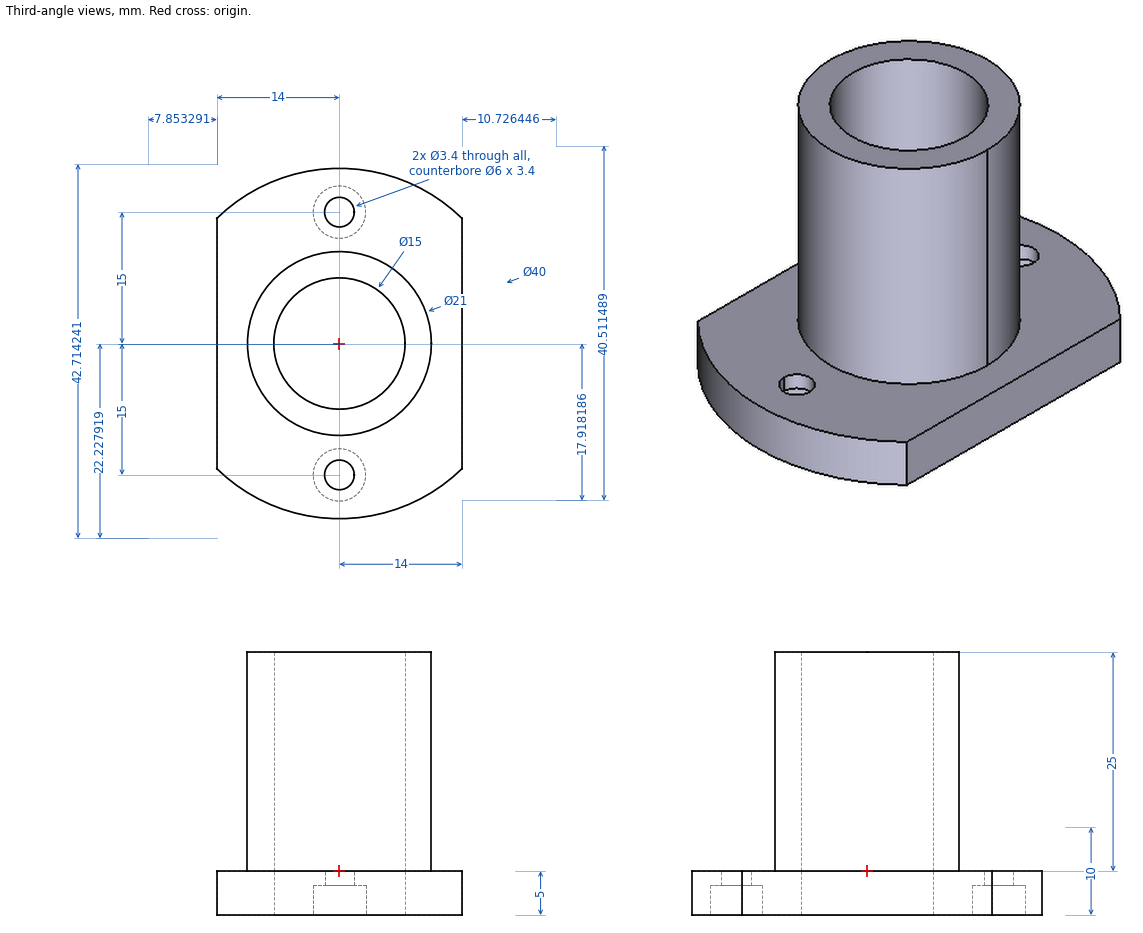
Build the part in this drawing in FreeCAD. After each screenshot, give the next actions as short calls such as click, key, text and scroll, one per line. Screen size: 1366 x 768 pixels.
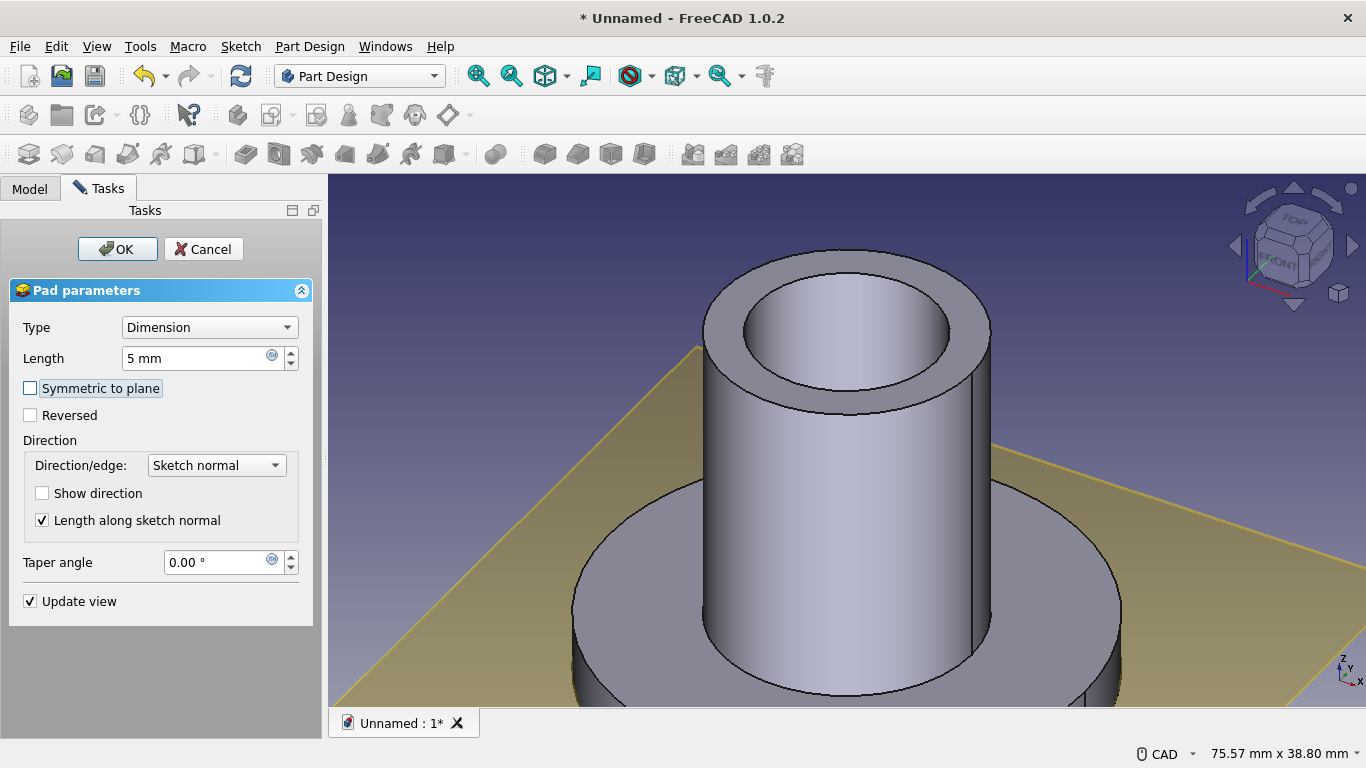
click(118, 249)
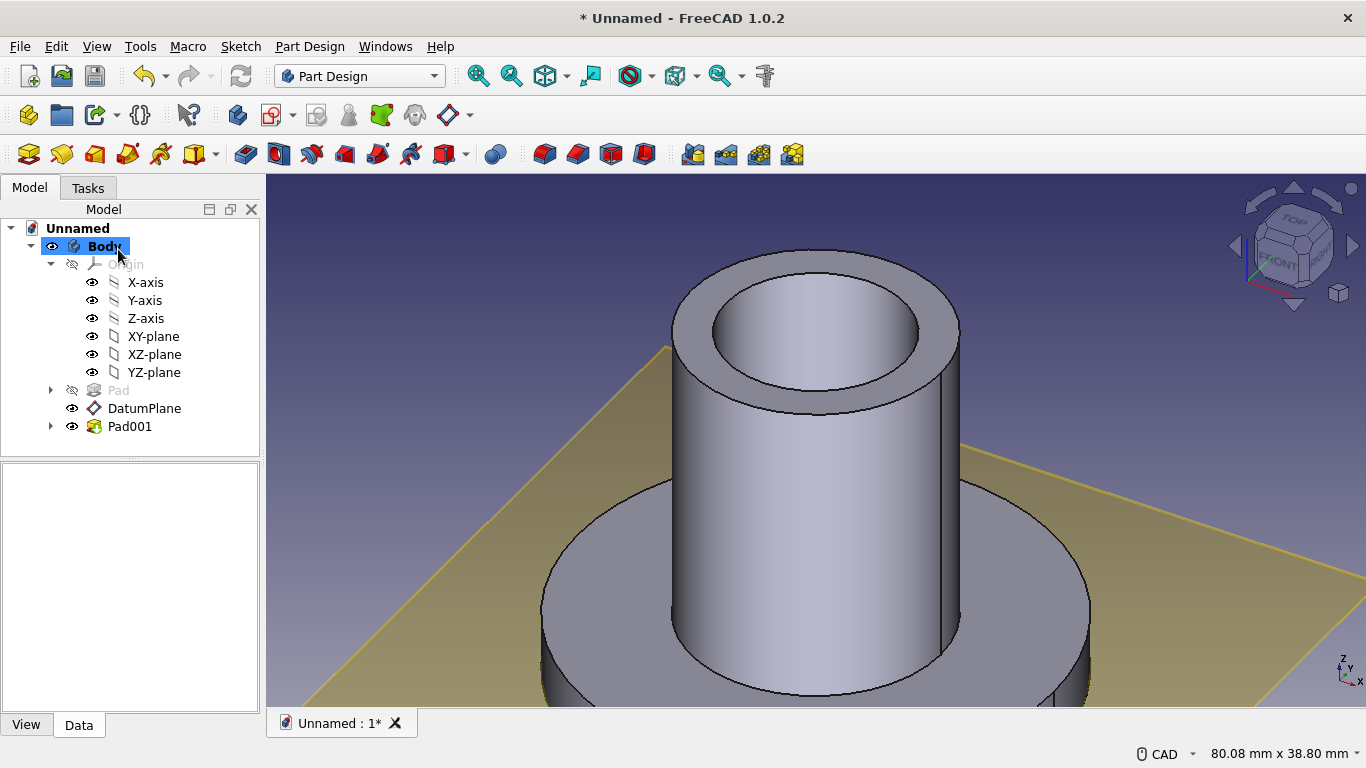
click(117, 408)
key(space)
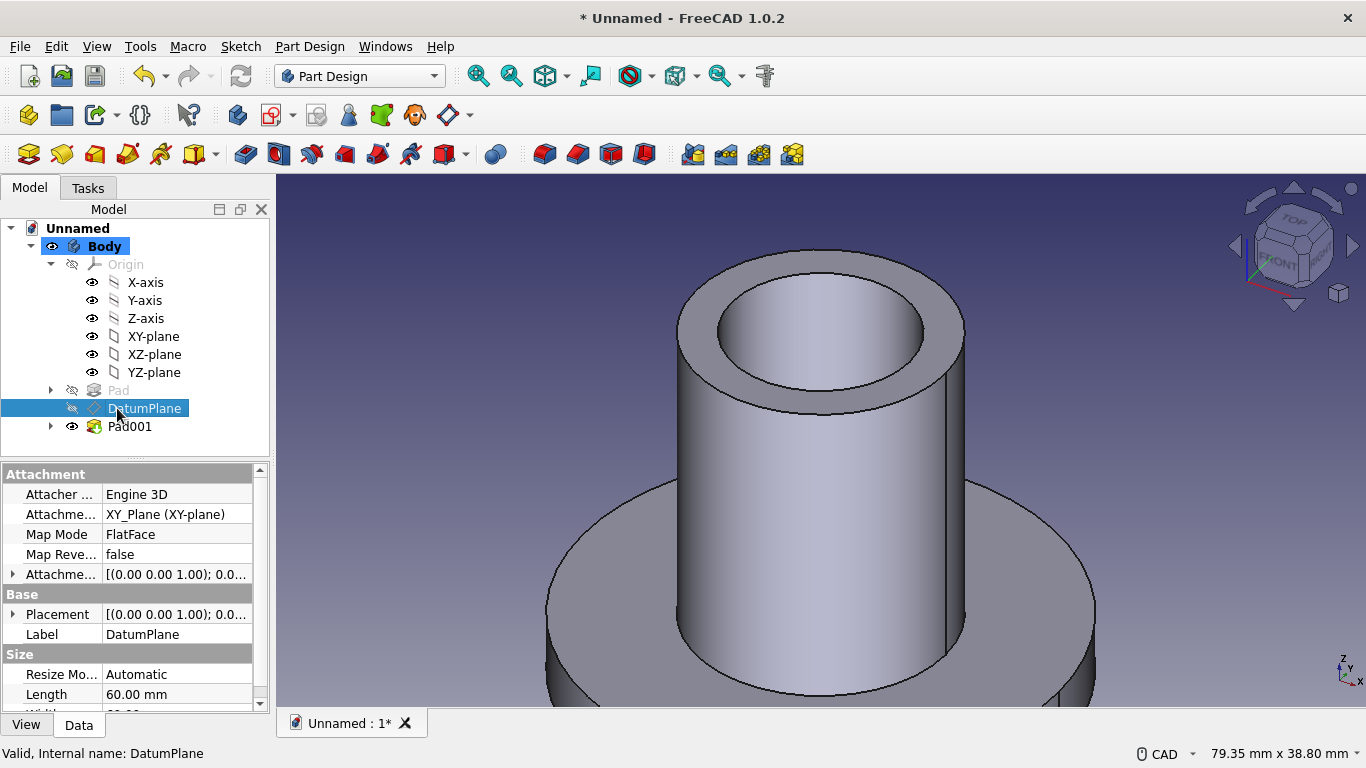
click(479, 76)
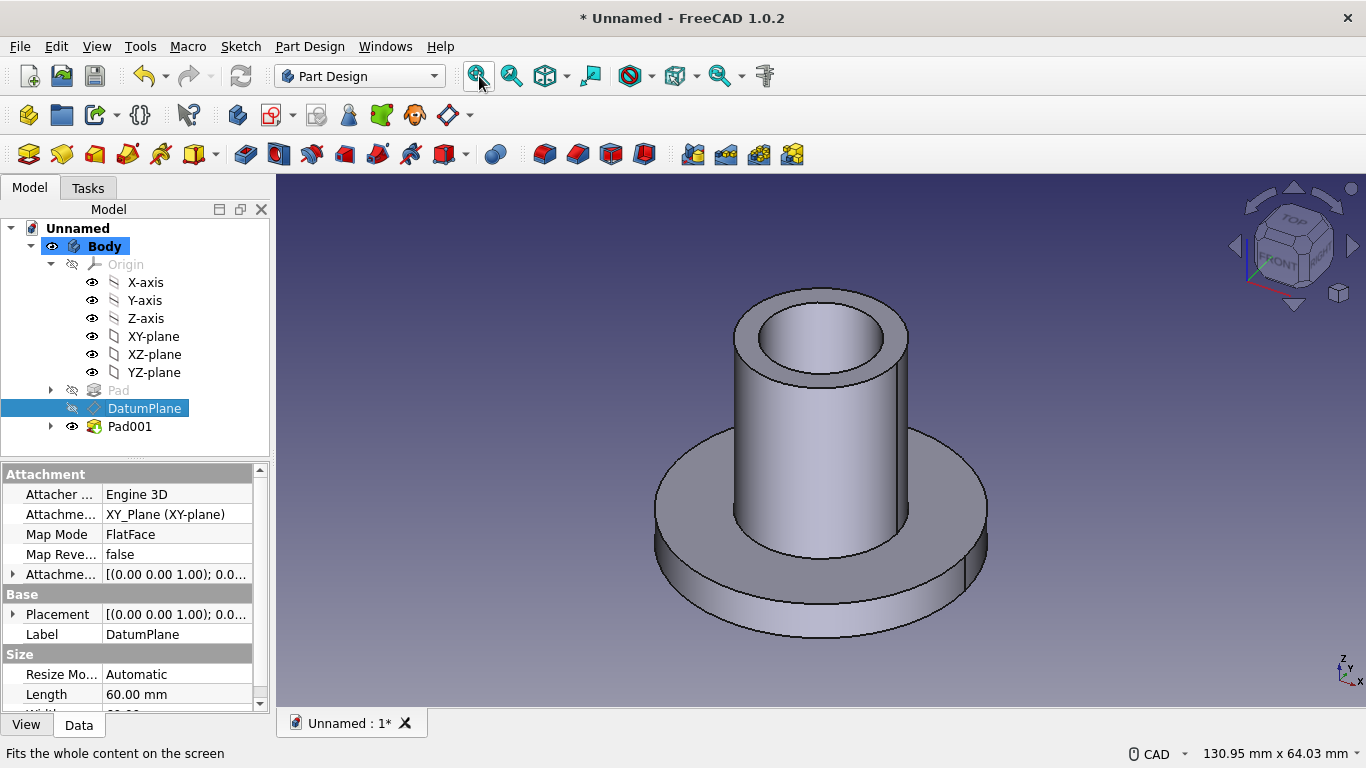
key(5)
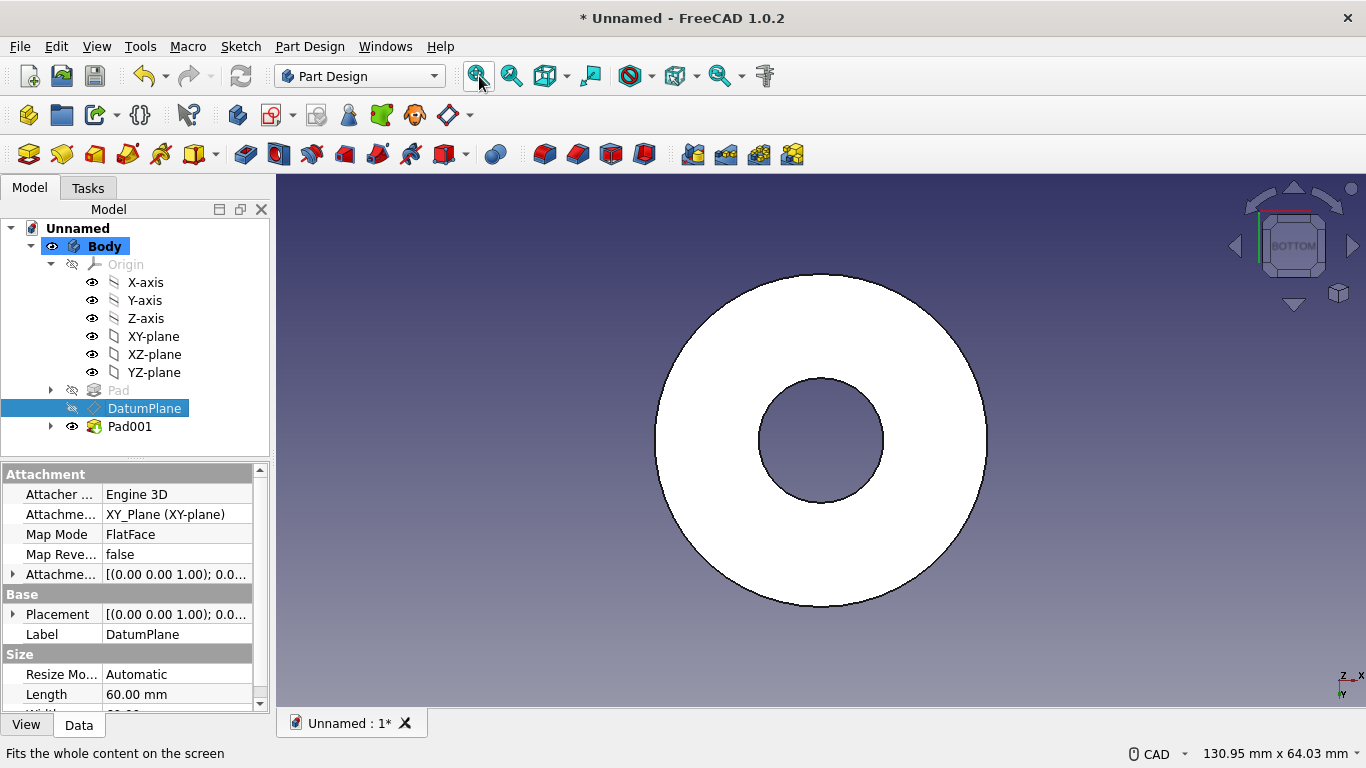
click(726, 487)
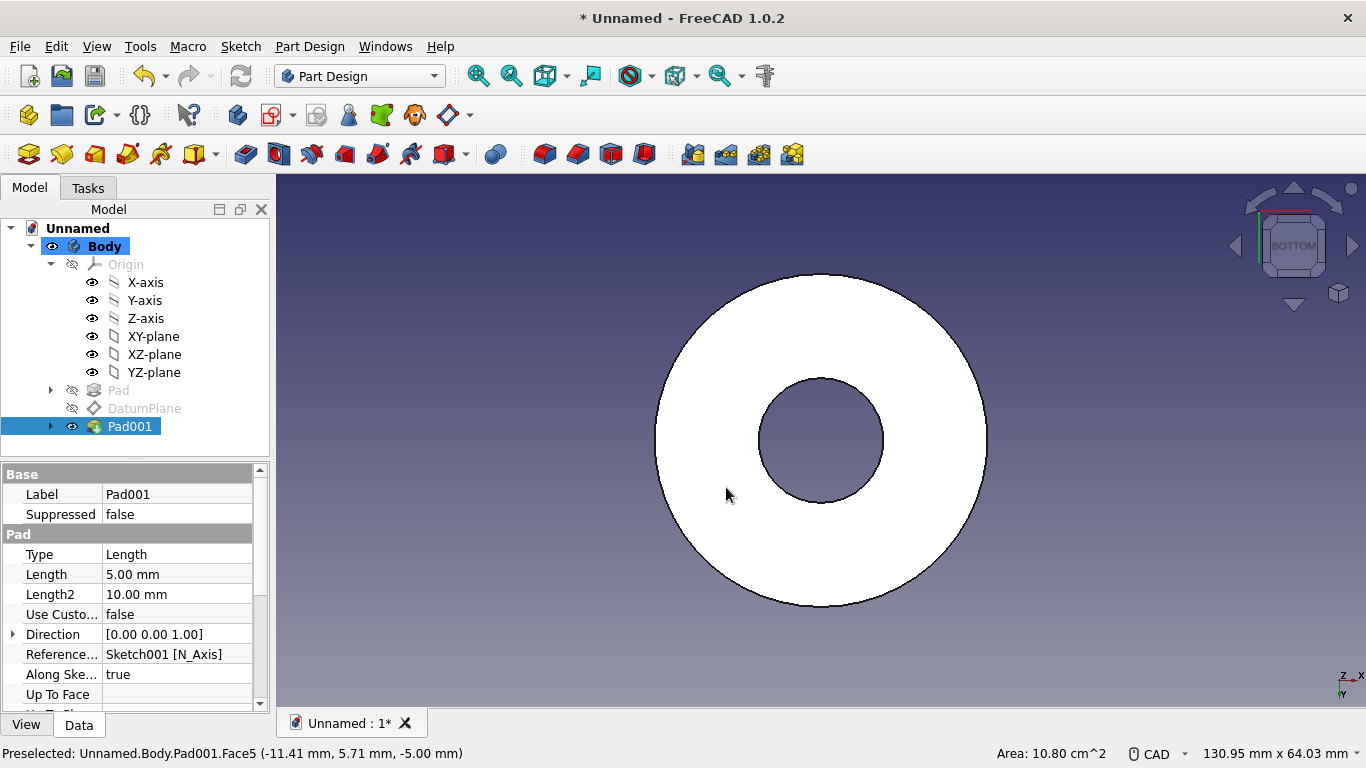
click(270, 116)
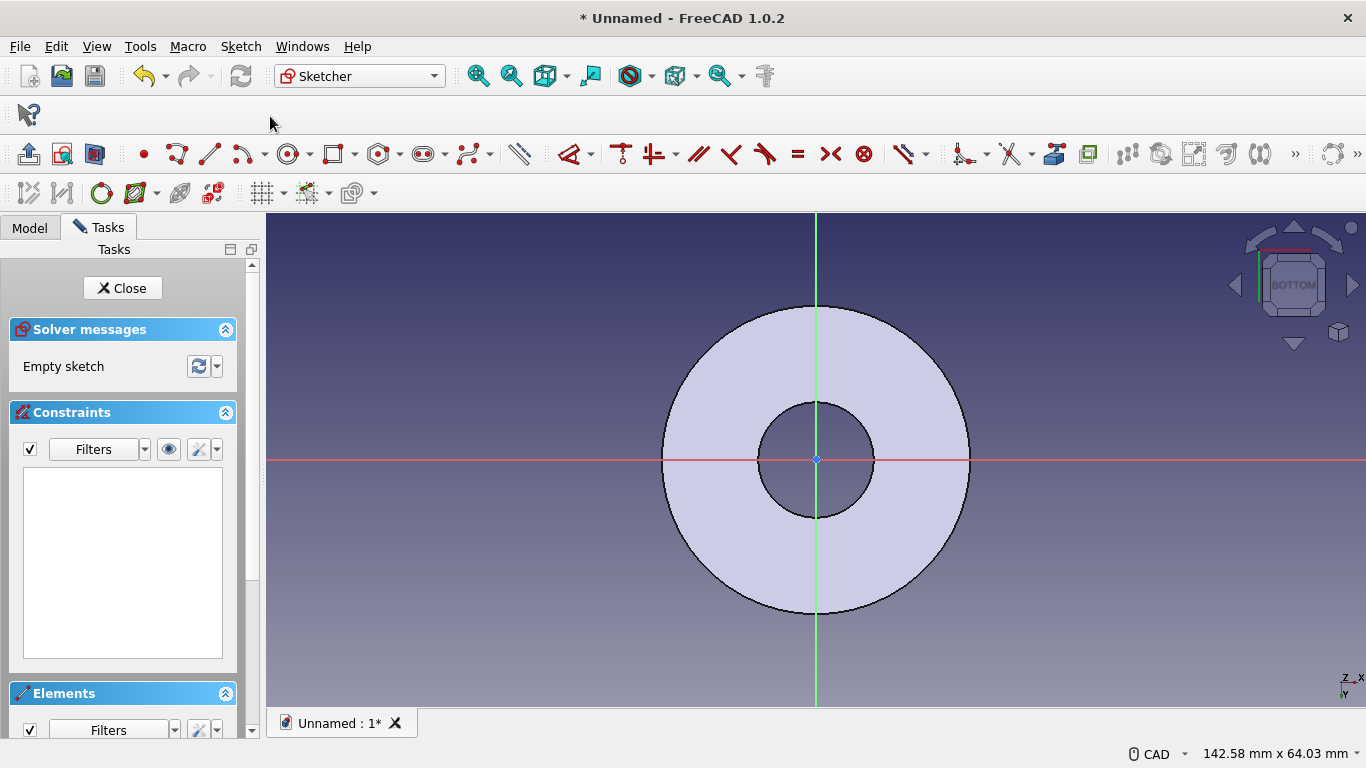
click(288, 154)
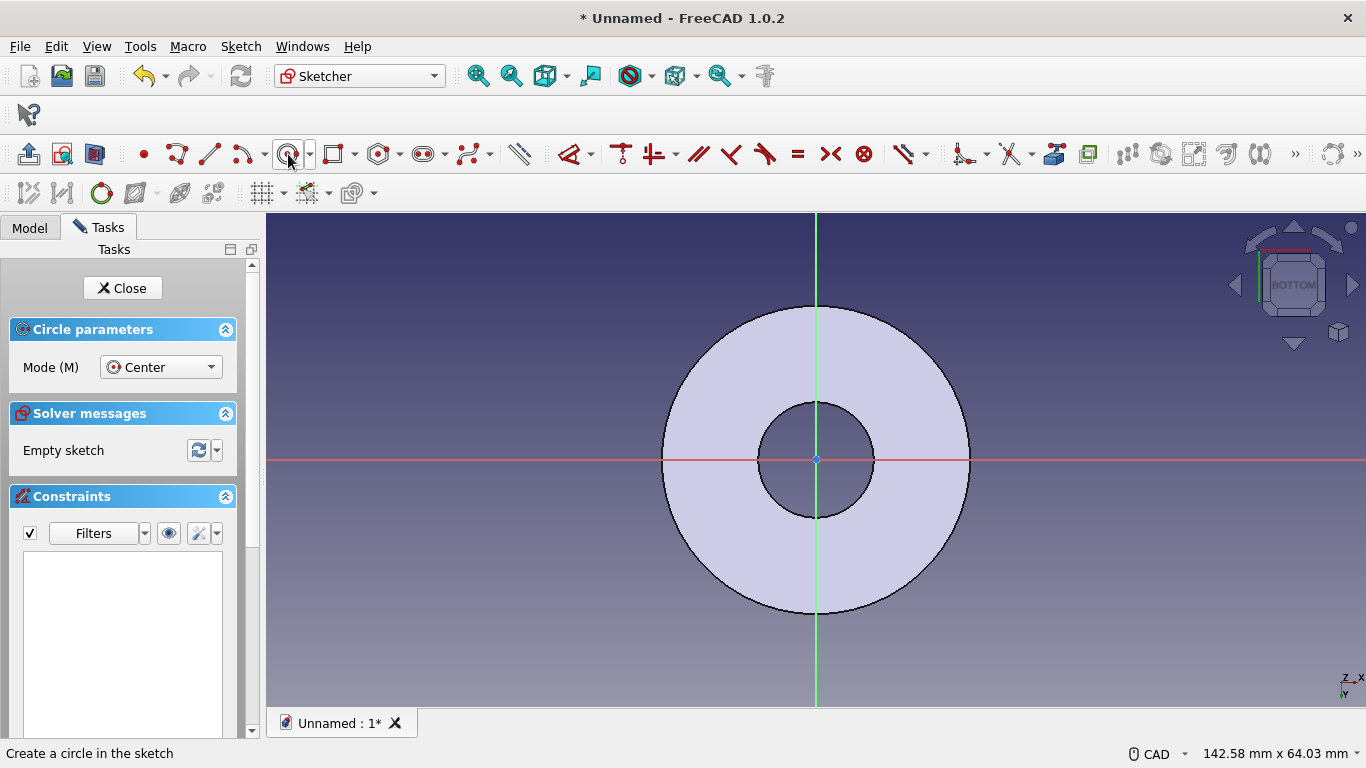
scroll(816, 576, up, 3)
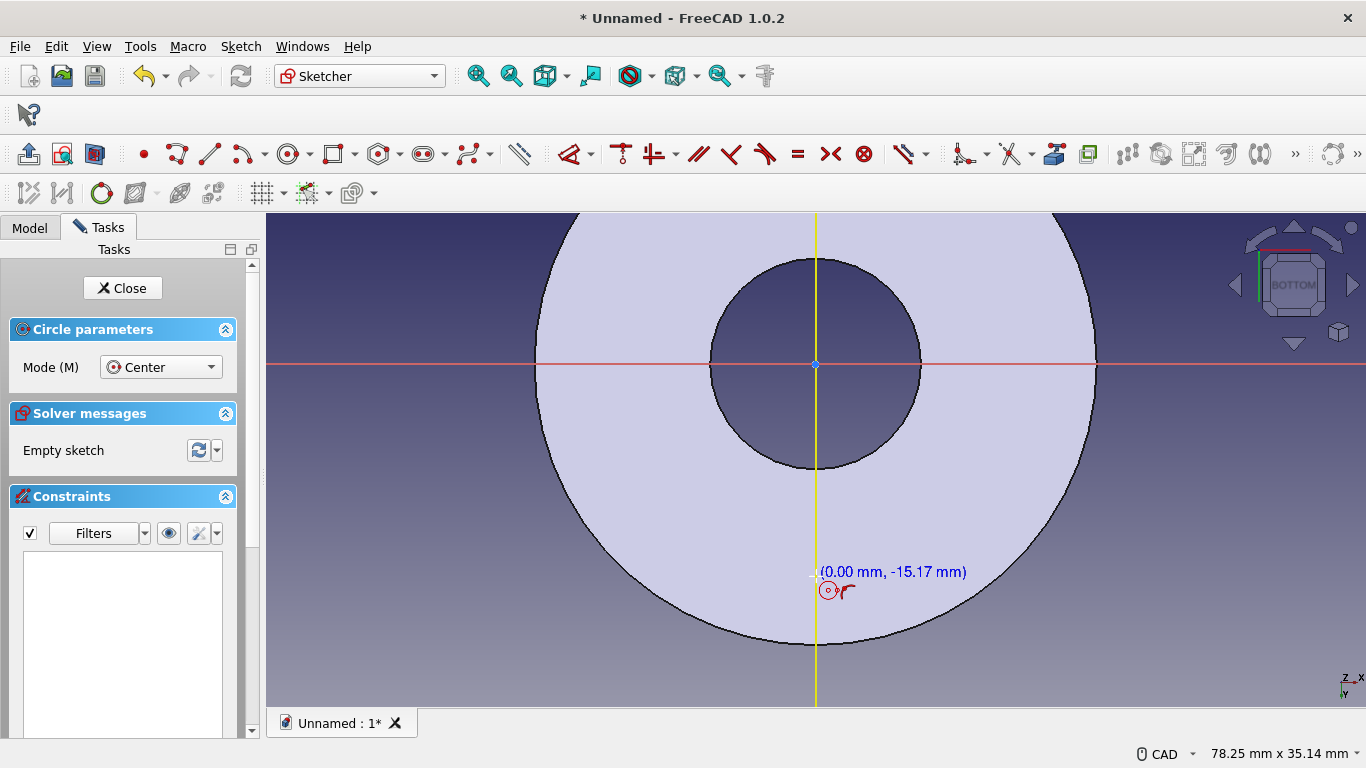
click(816, 575)
move(832, 558)